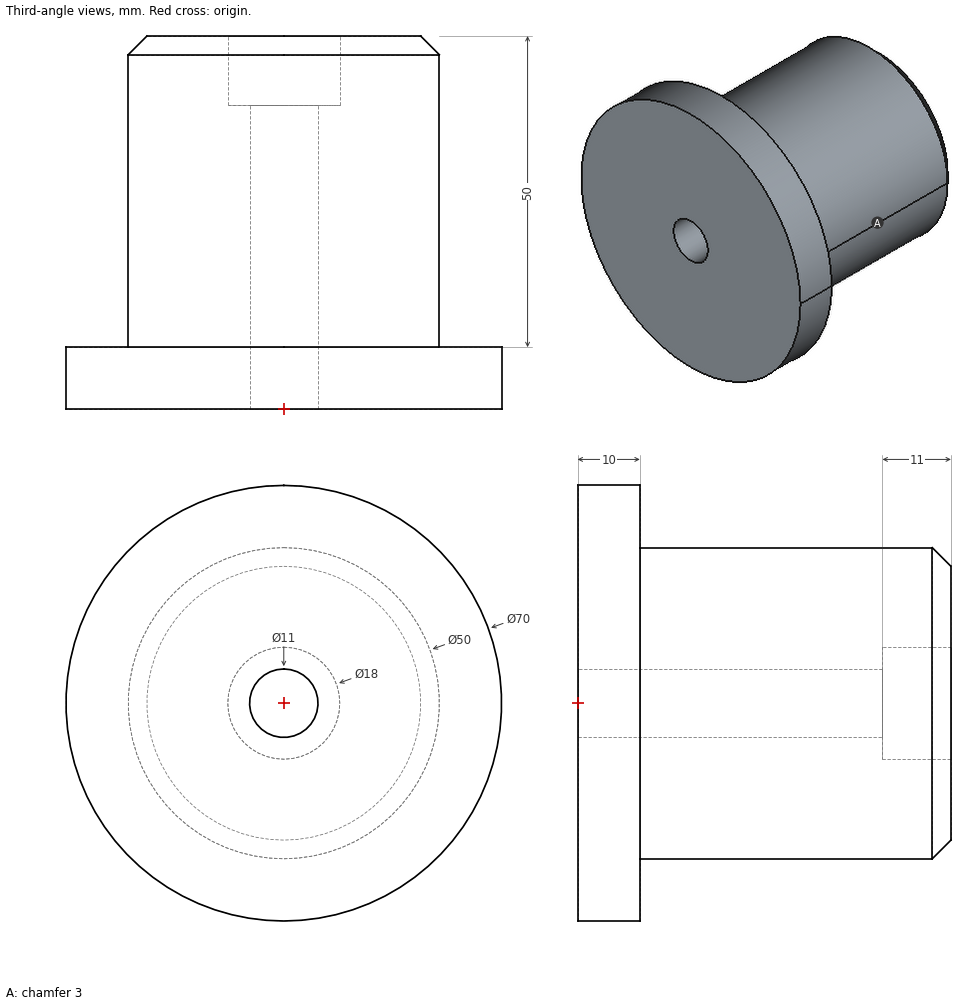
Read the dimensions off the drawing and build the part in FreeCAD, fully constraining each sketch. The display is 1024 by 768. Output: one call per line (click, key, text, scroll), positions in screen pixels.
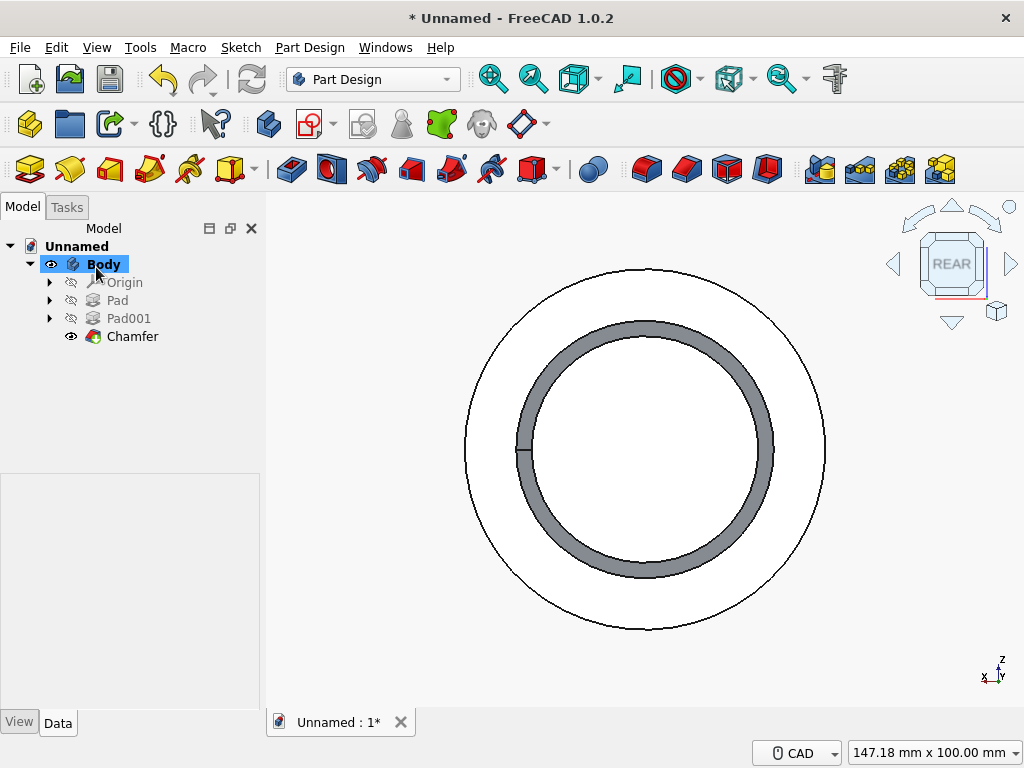
click(645, 448)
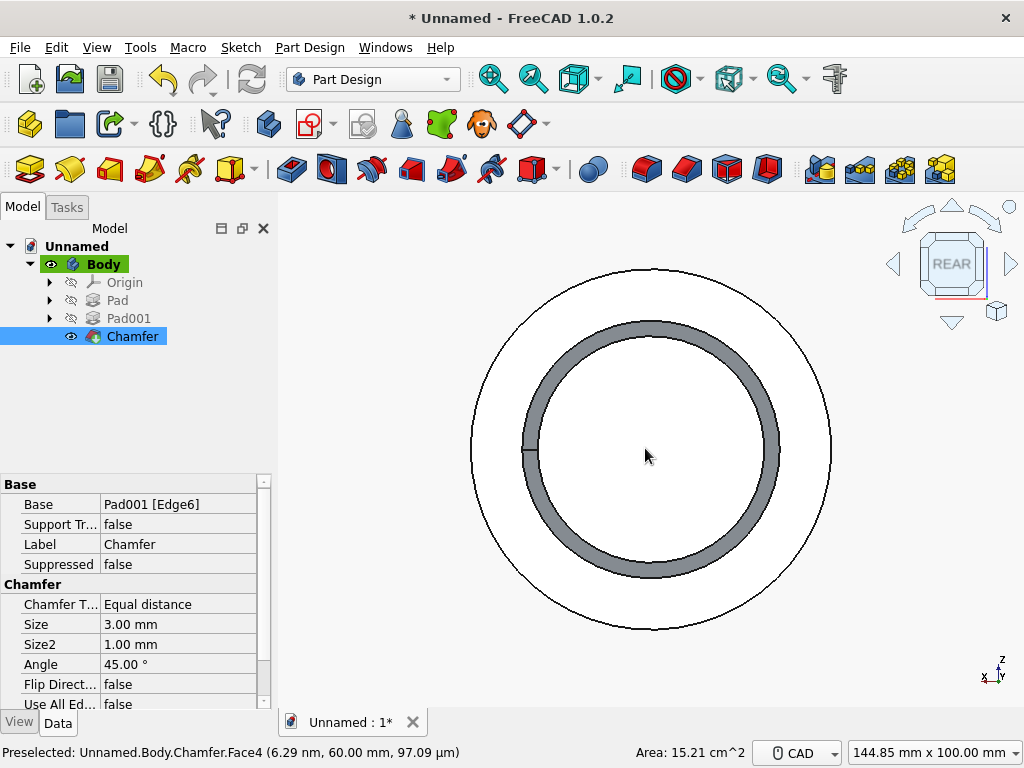
click(310, 124)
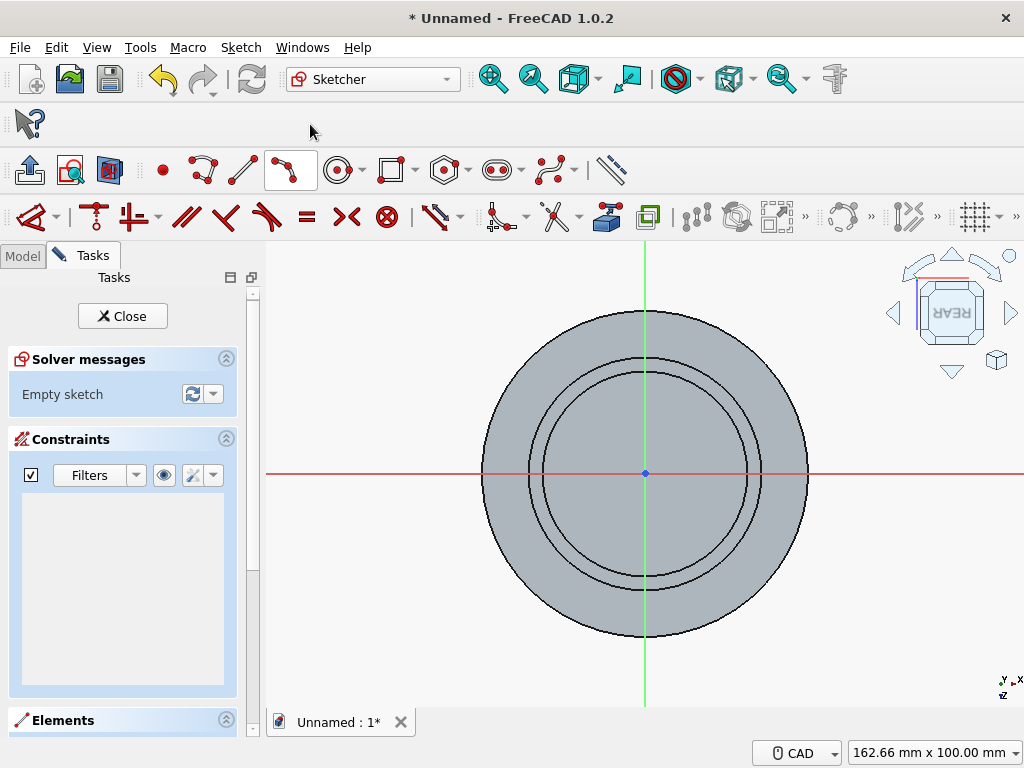
scroll(675, 474, up, 6)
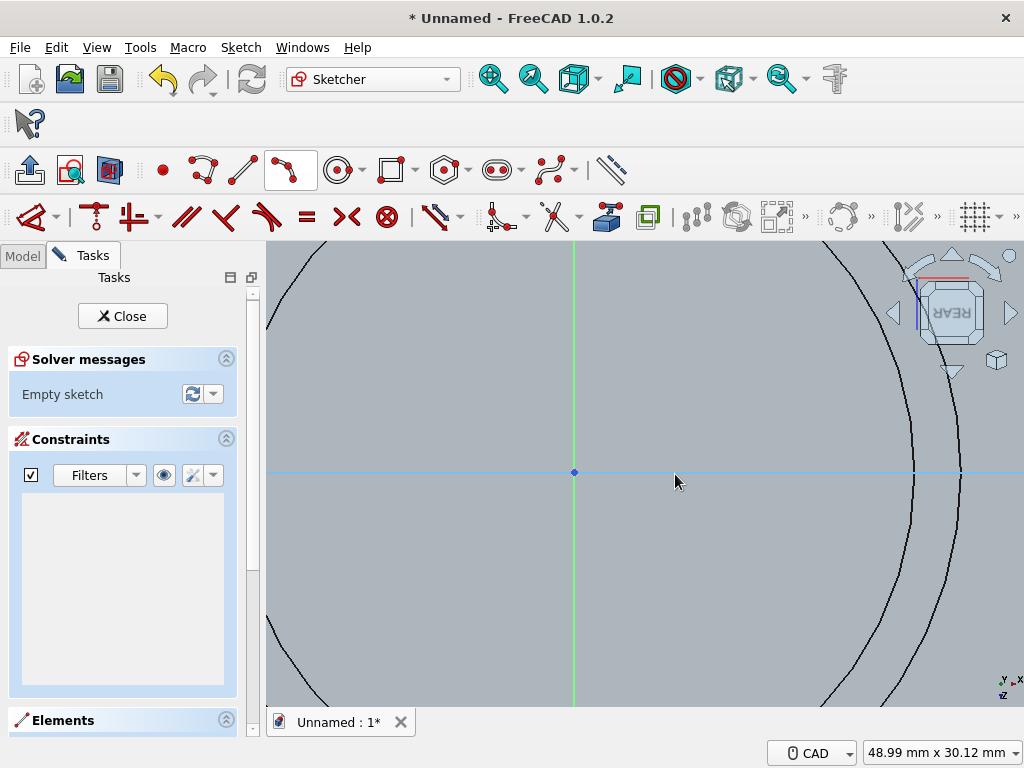
key(g)
key(c)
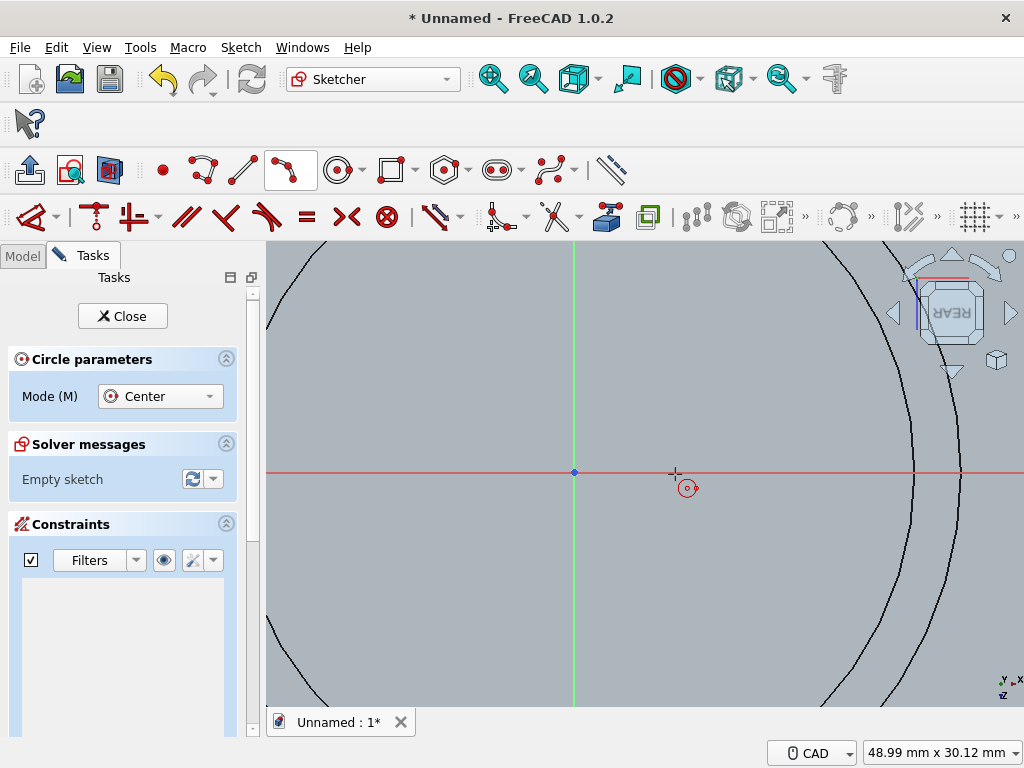
click(574, 473)
move(673, 374)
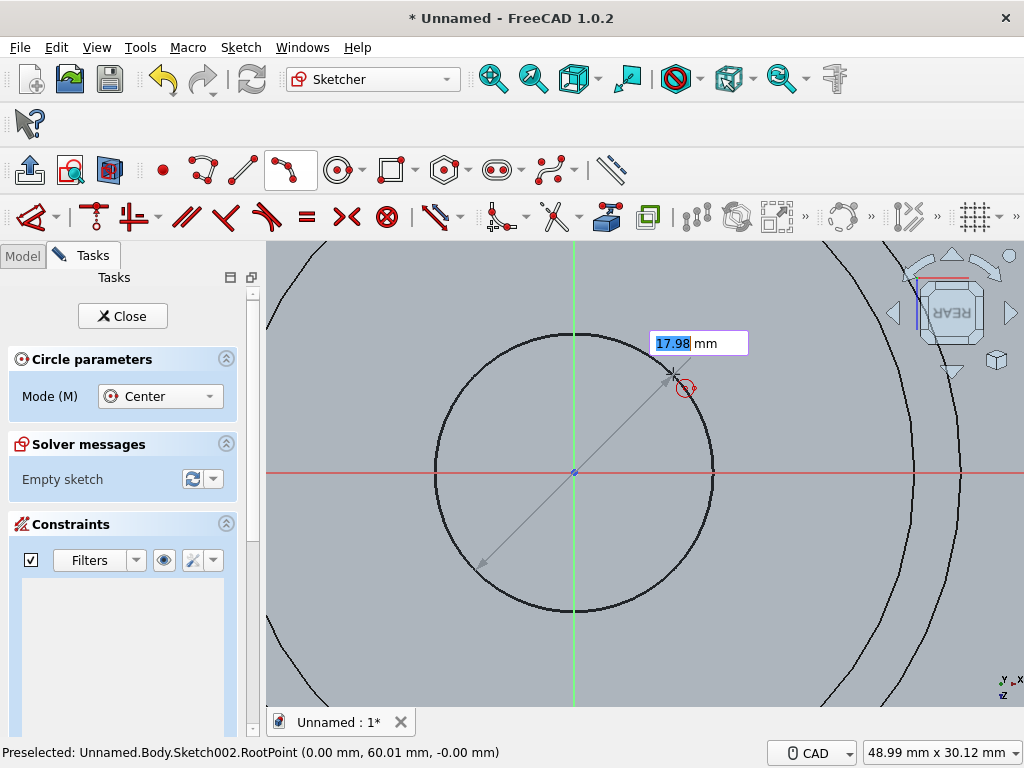
text(18)
key(Return)
key(Escape)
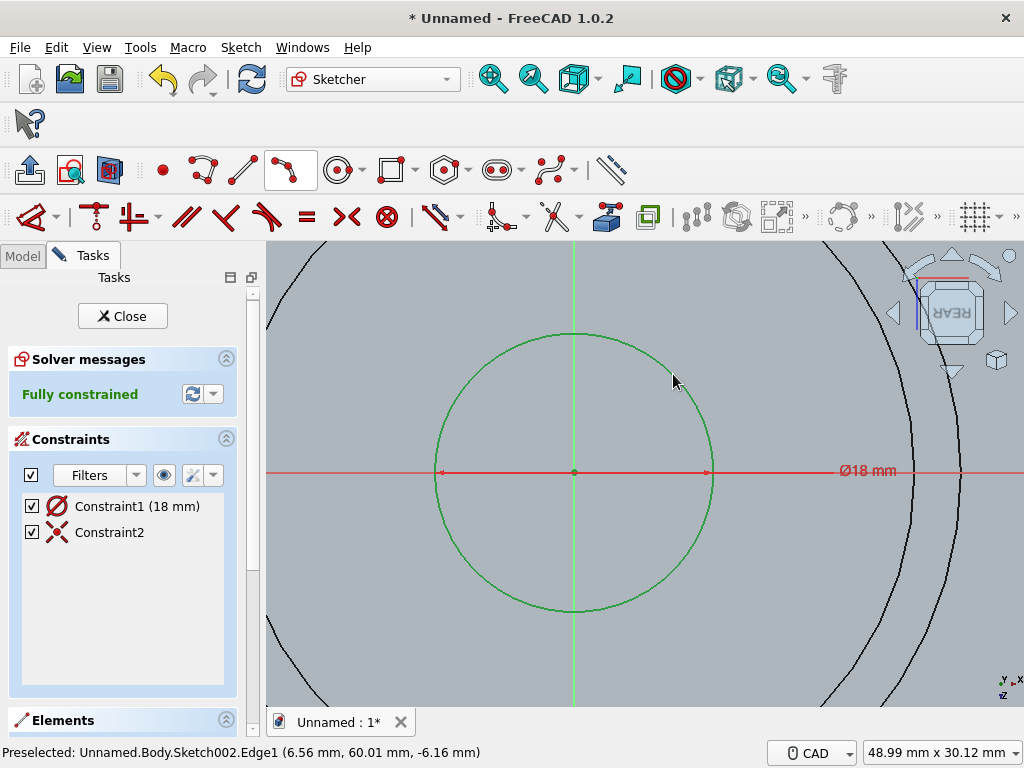
click(123, 316)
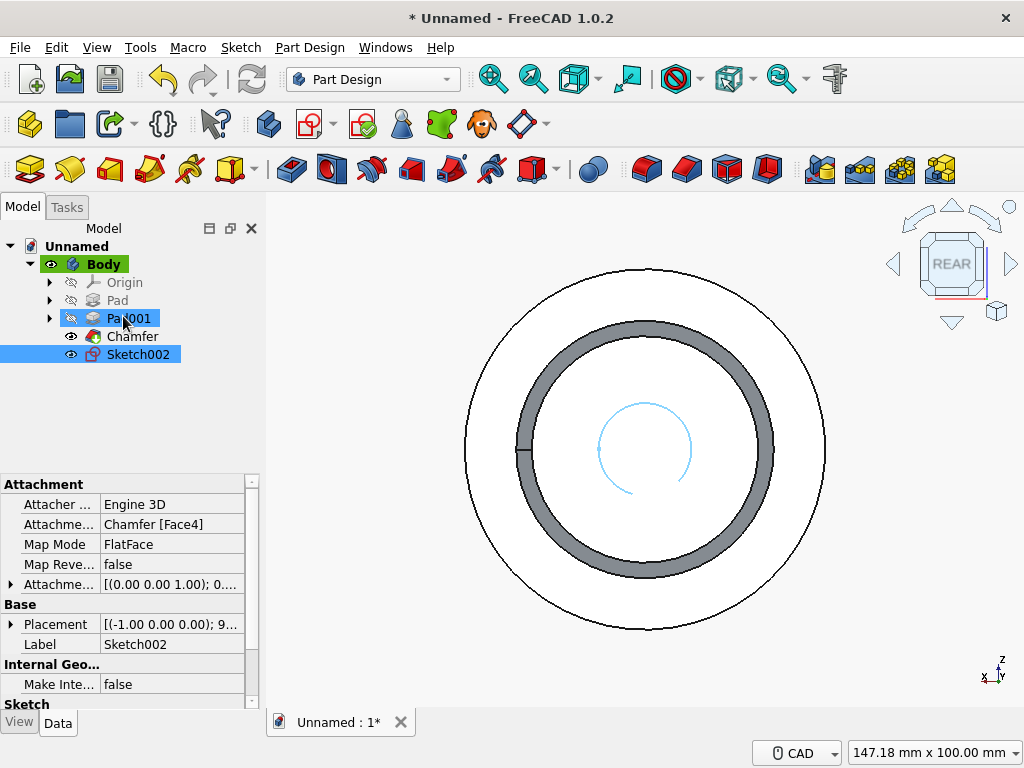
click(292, 170)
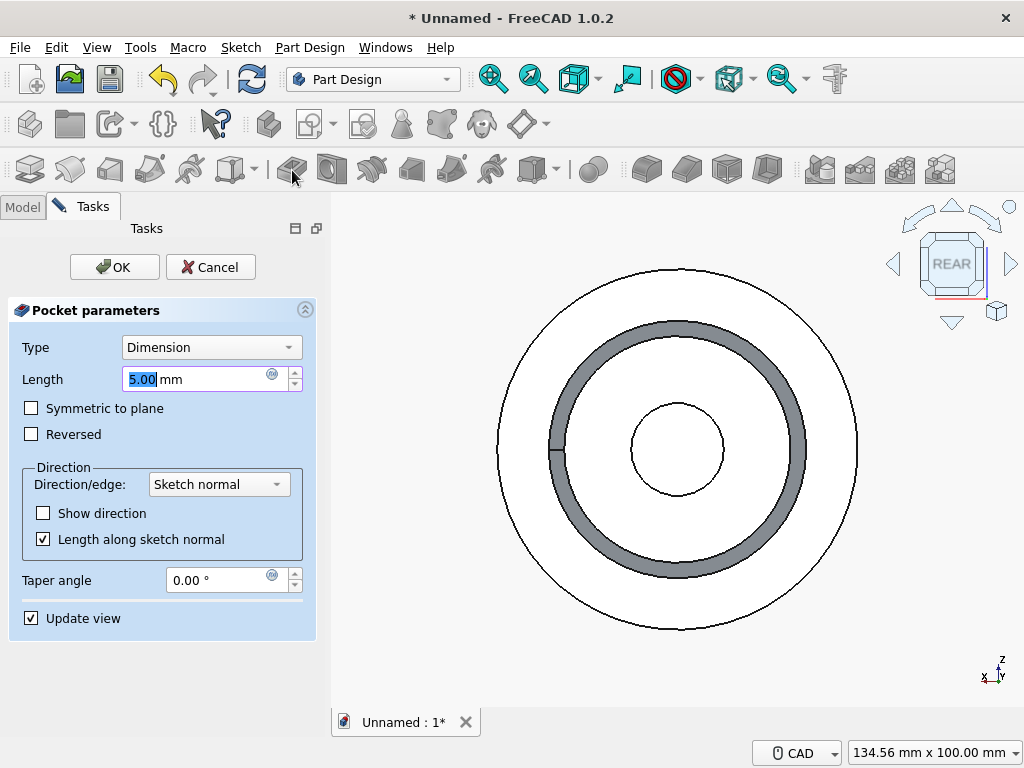
text(11)
key(Tab)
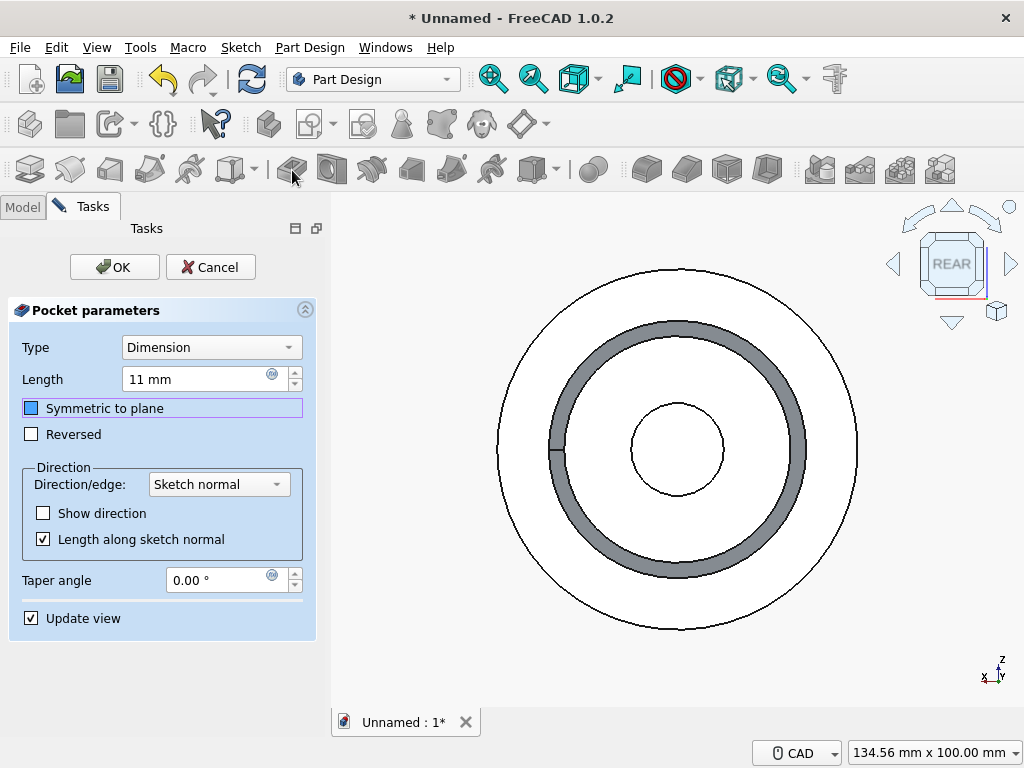
click(115, 267)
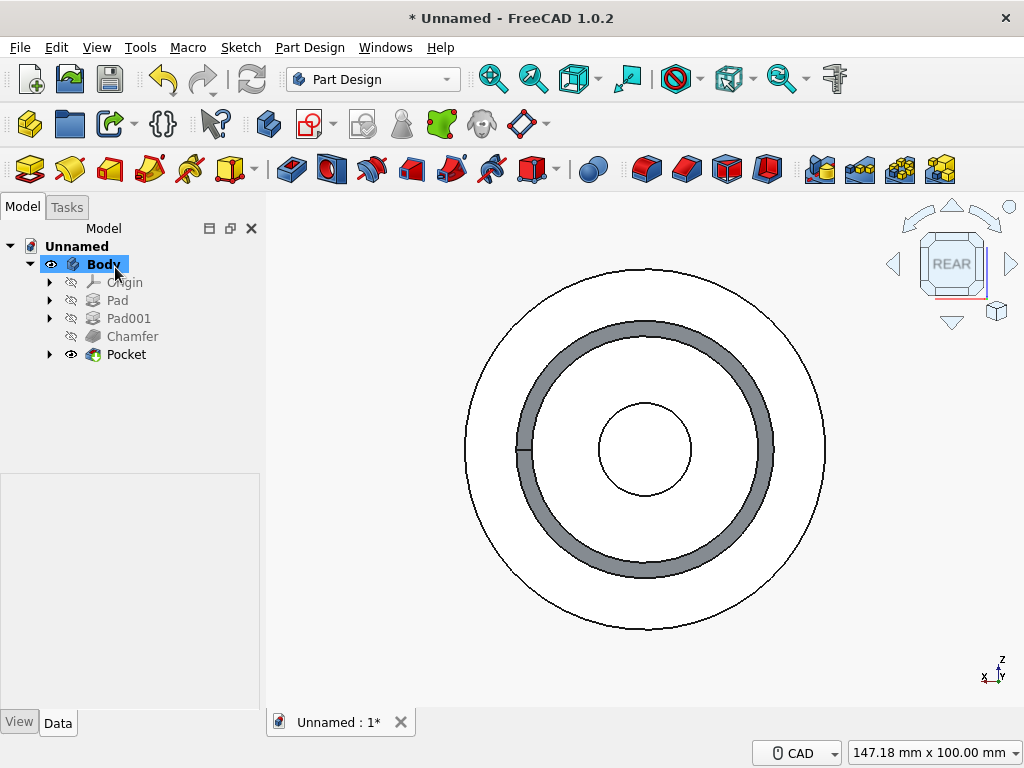
click(645, 448)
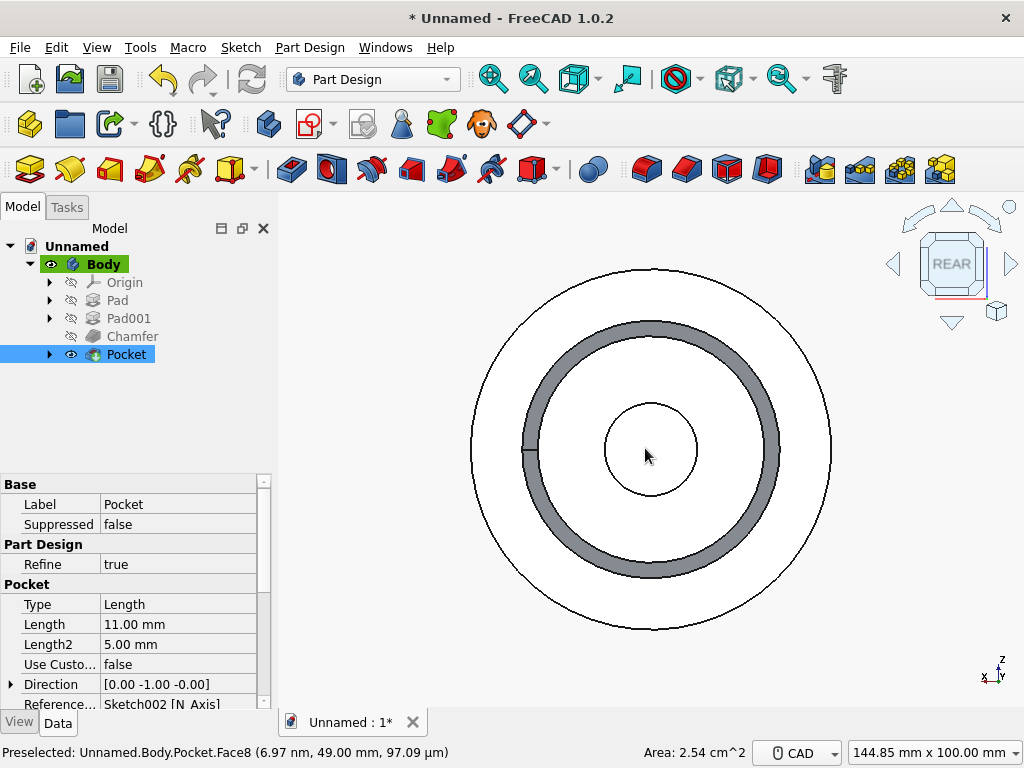
click(310, 124)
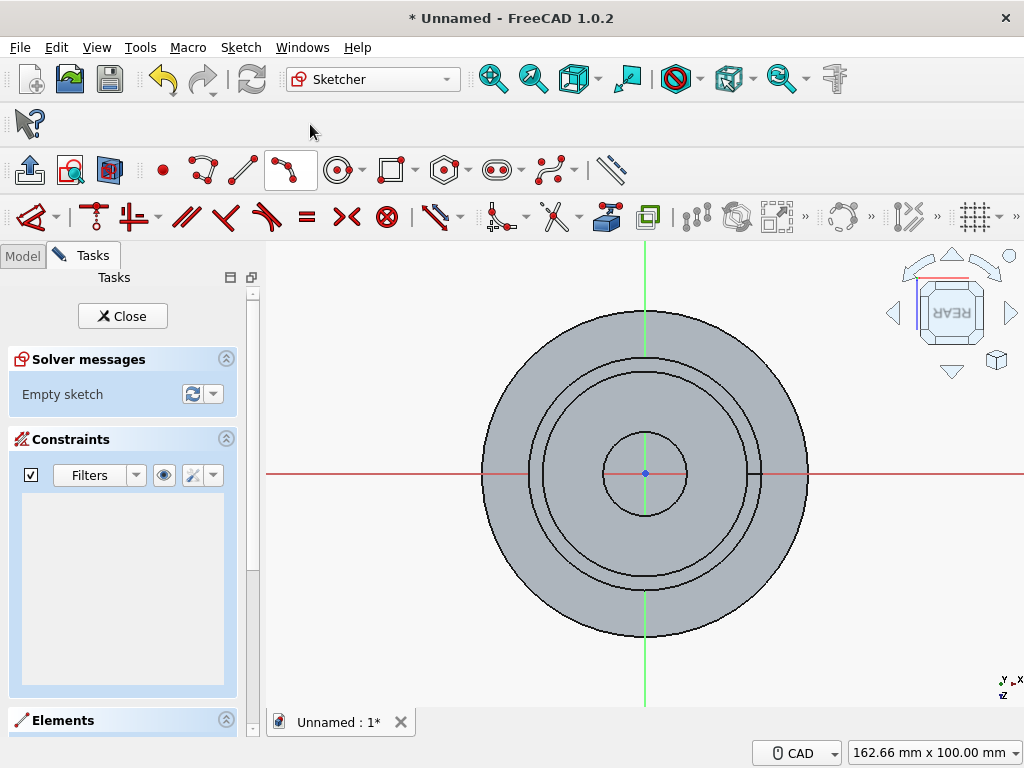
scroll(659, 474, up, 9)